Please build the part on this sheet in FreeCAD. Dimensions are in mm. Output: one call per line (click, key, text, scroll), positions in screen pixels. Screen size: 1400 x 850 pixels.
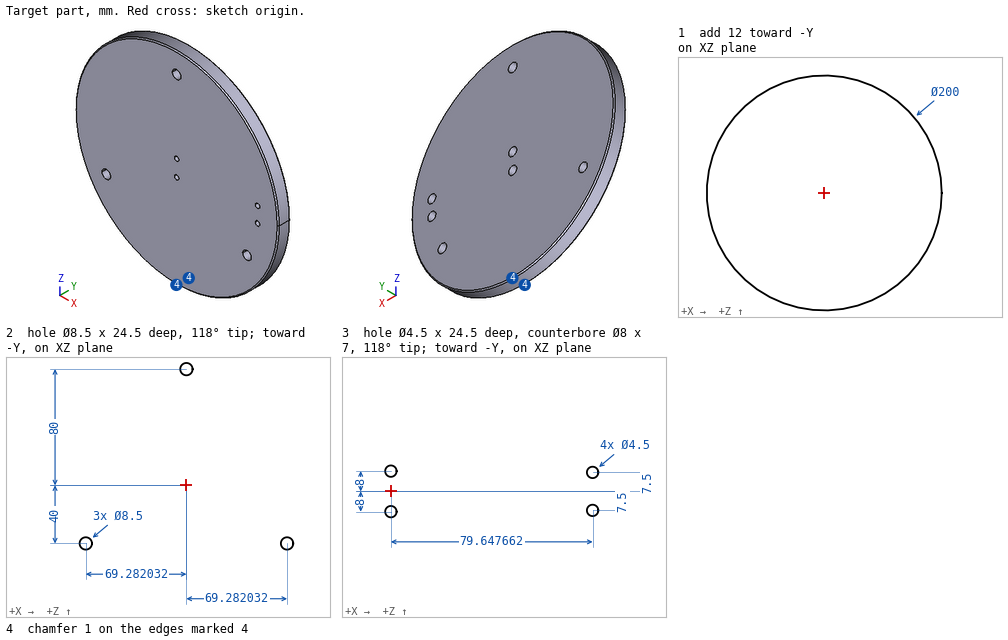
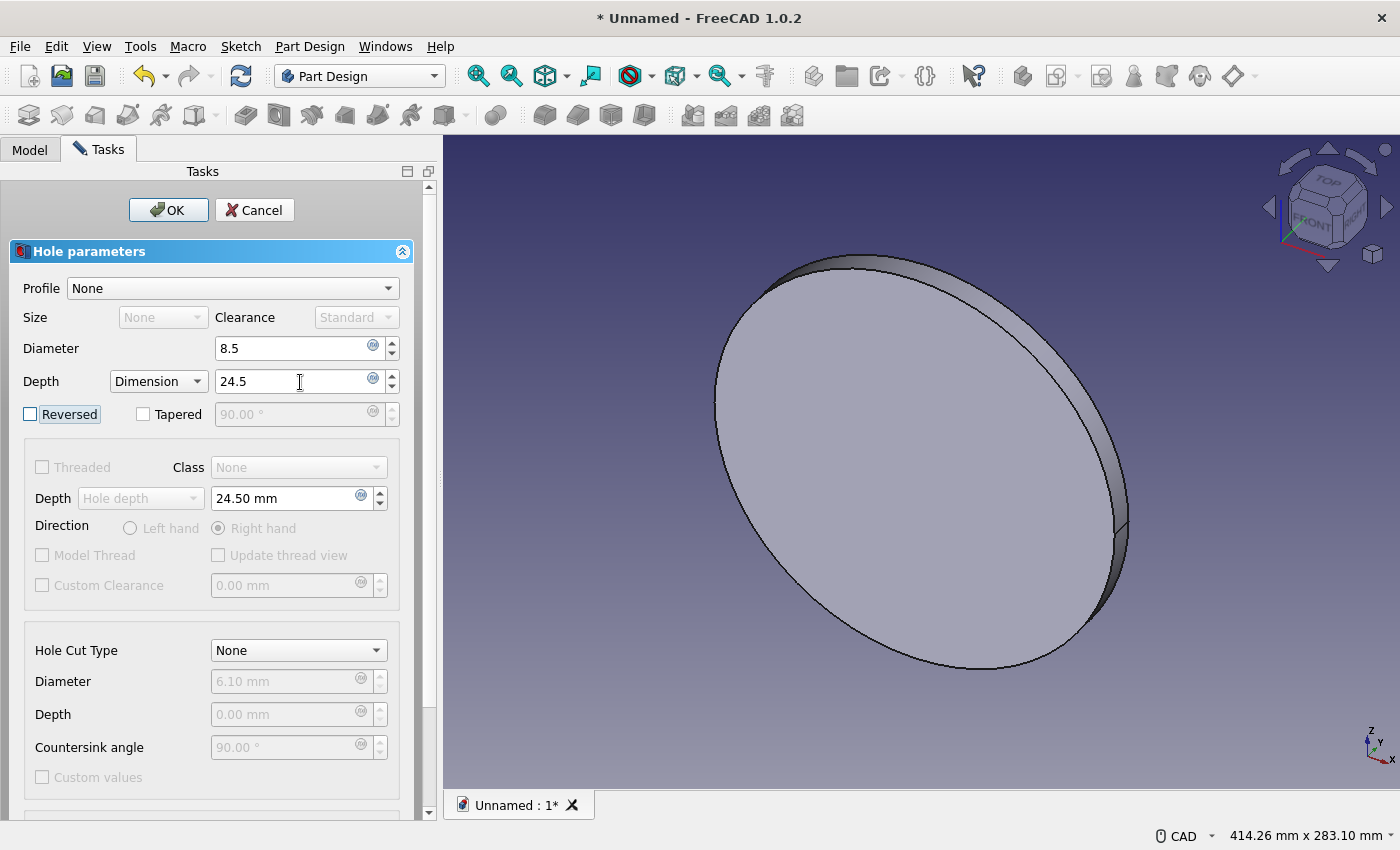
click(31, 414)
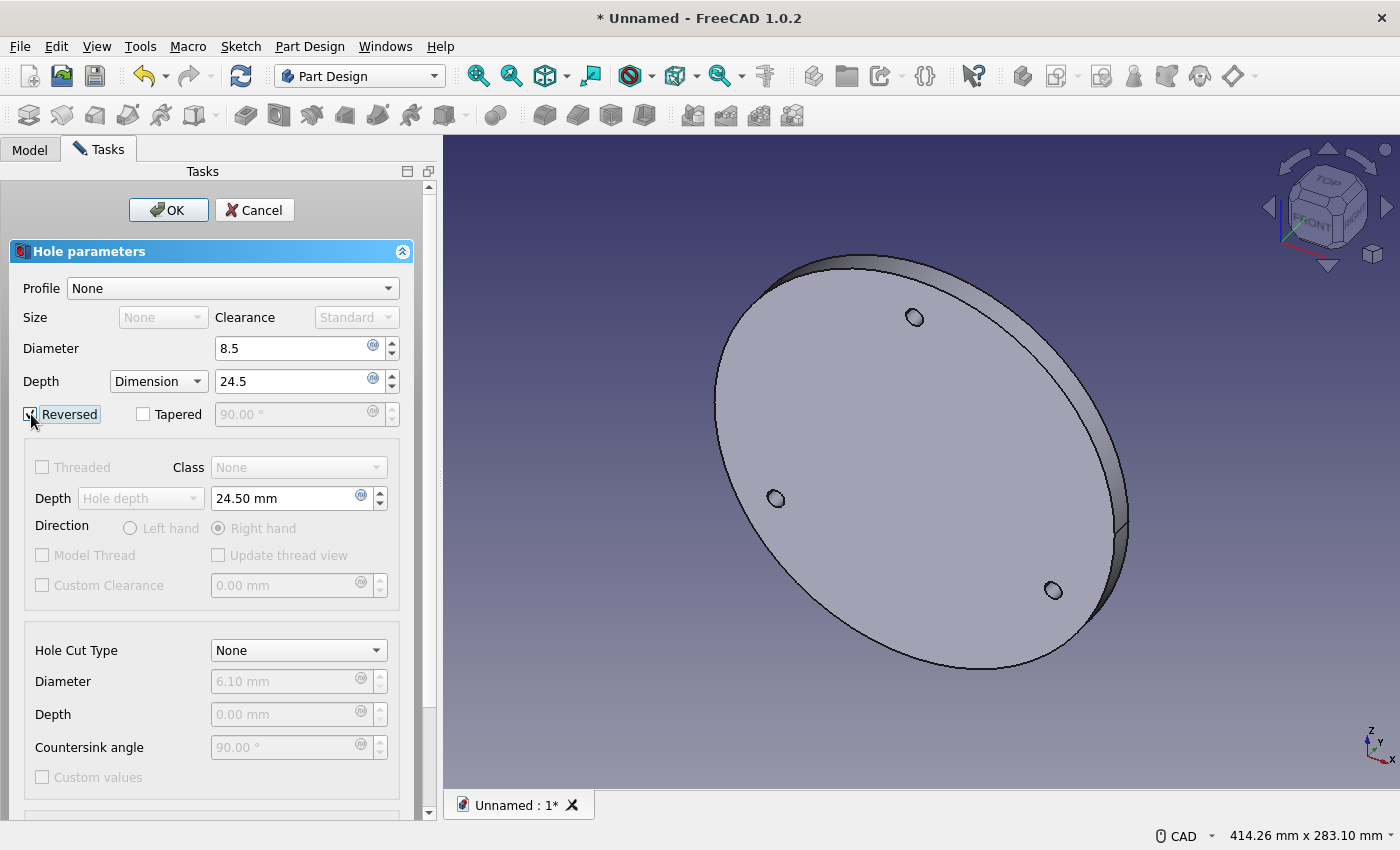
click(169, 210)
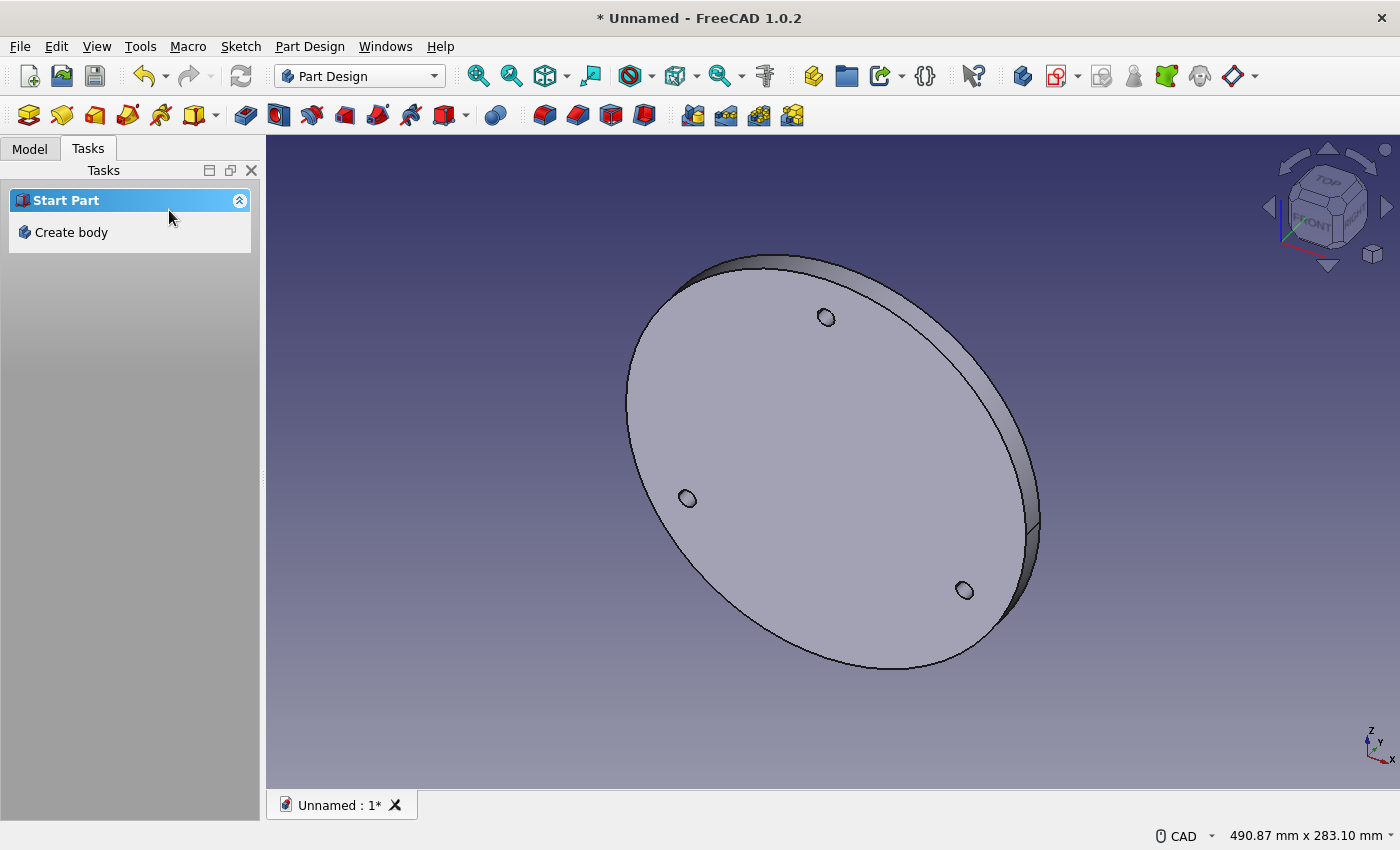
click(1056, 76)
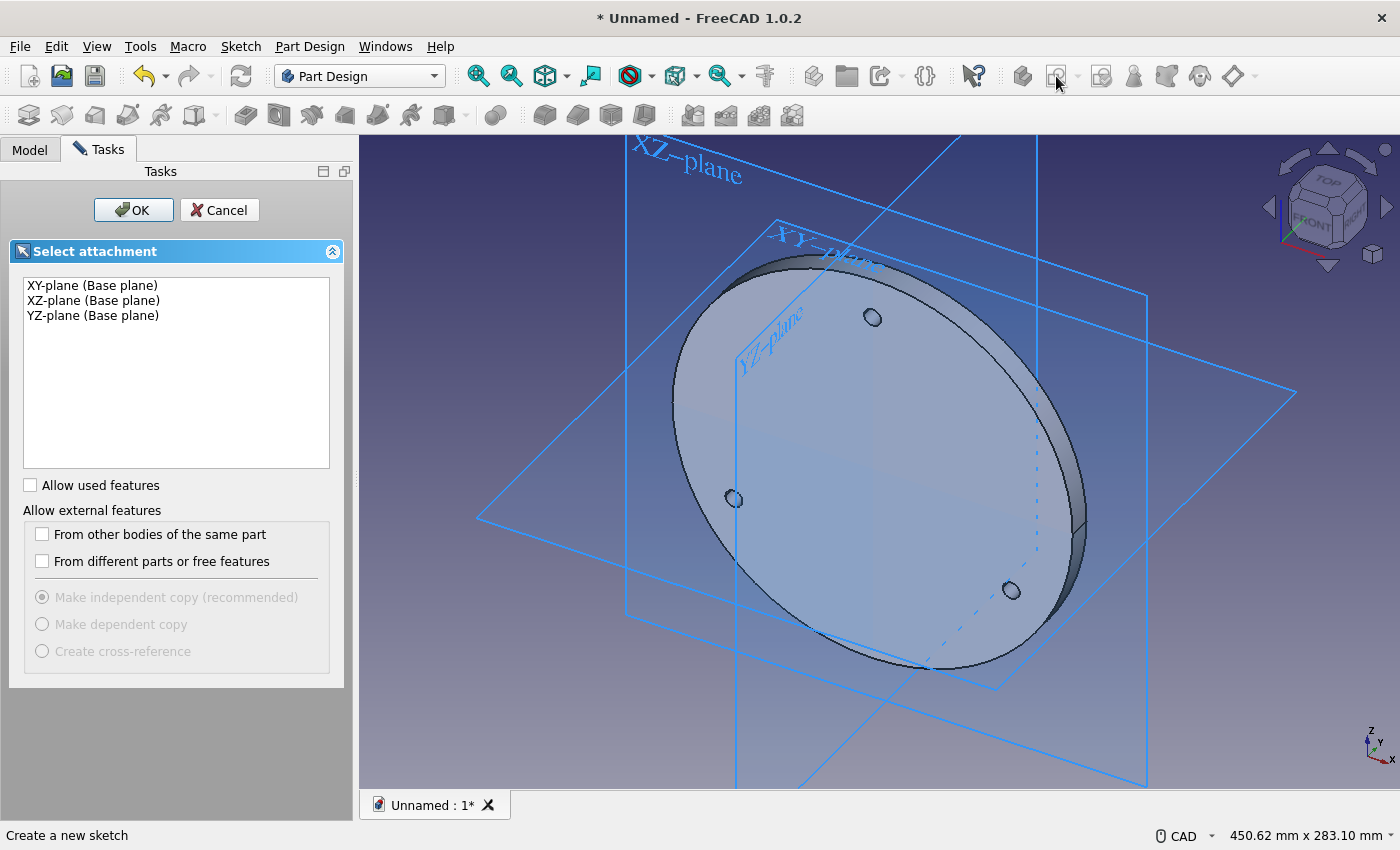
click(84, 300)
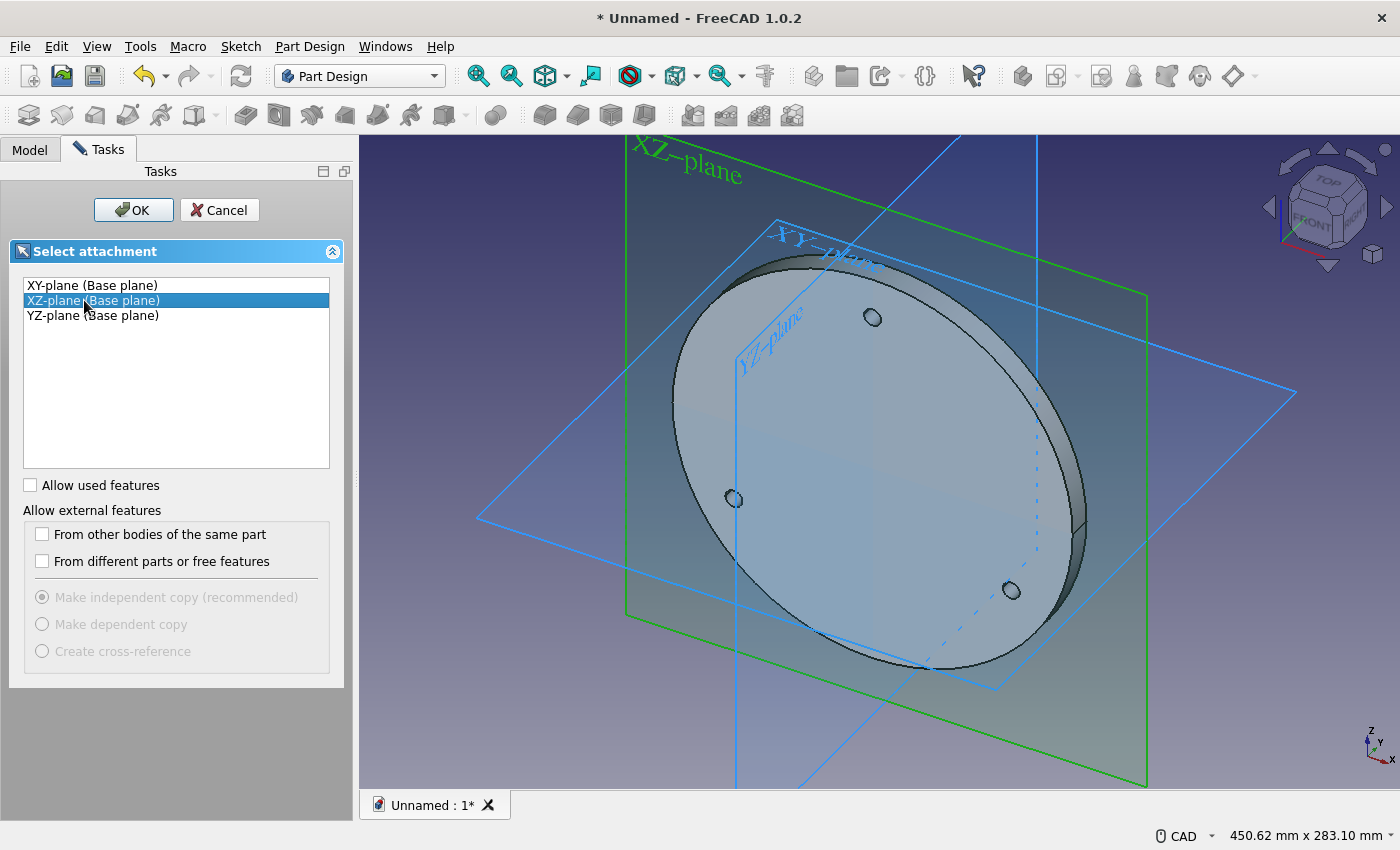
click(134, 210)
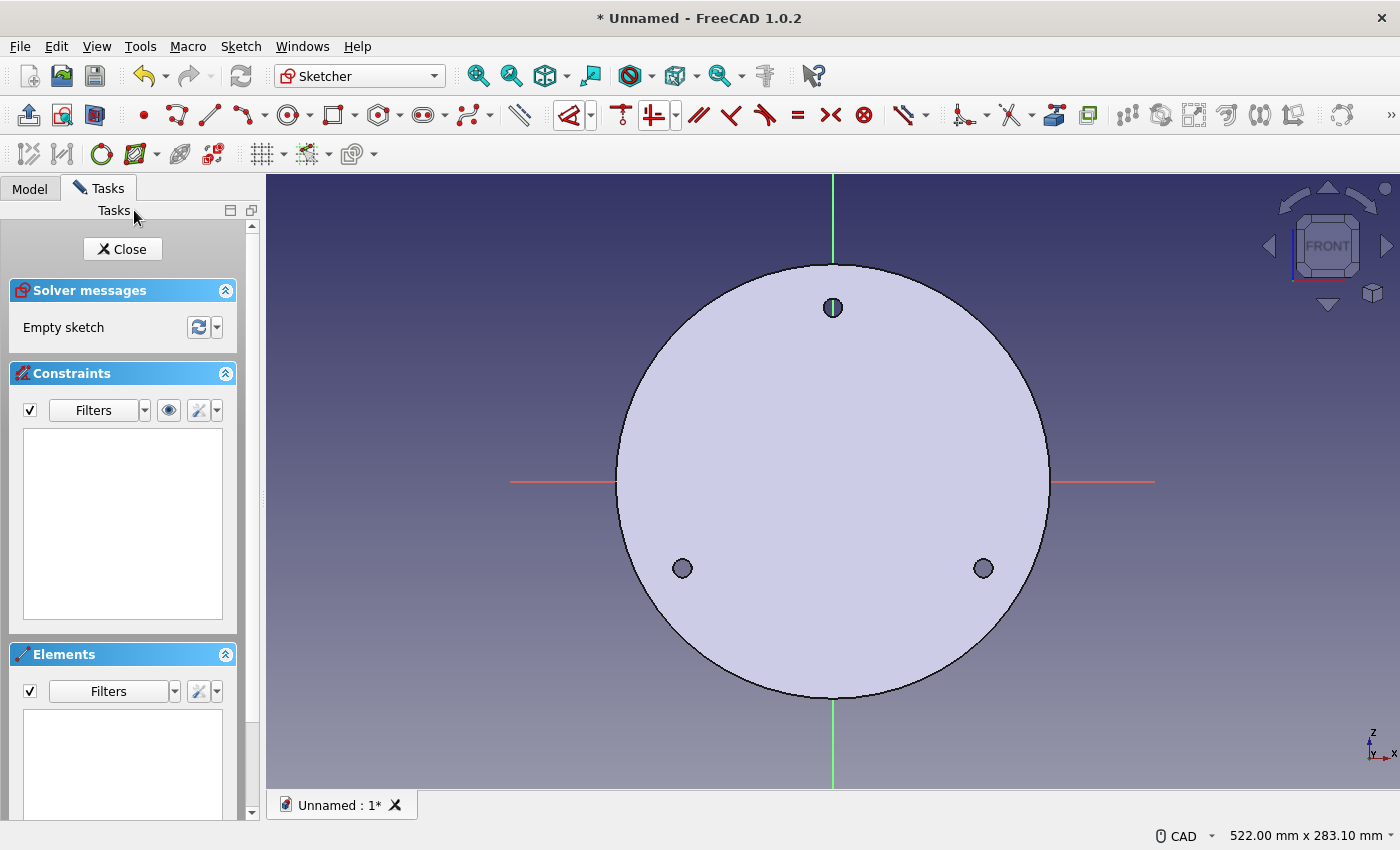
key(q)
key(s)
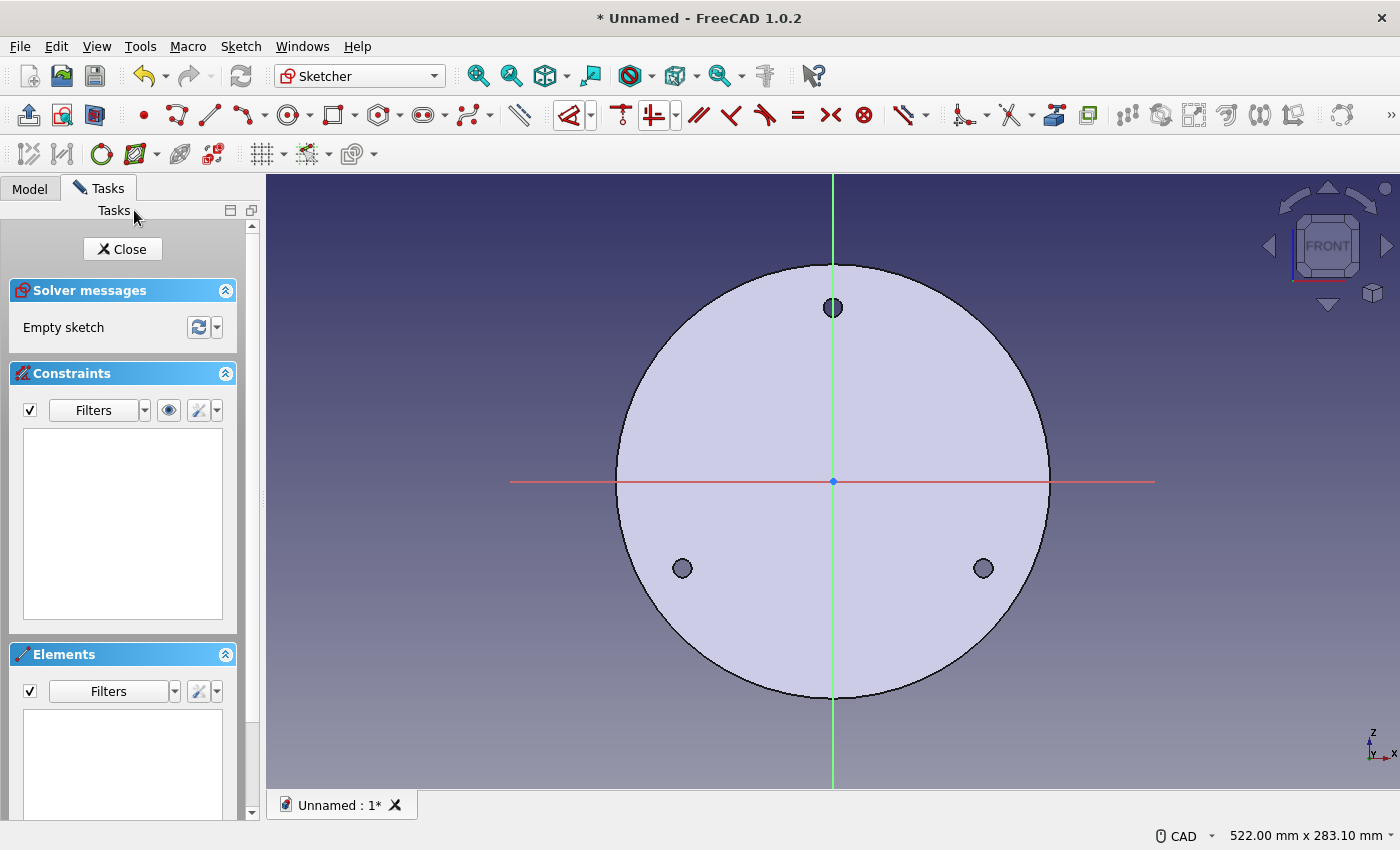
scroll(986, 482, up, 6)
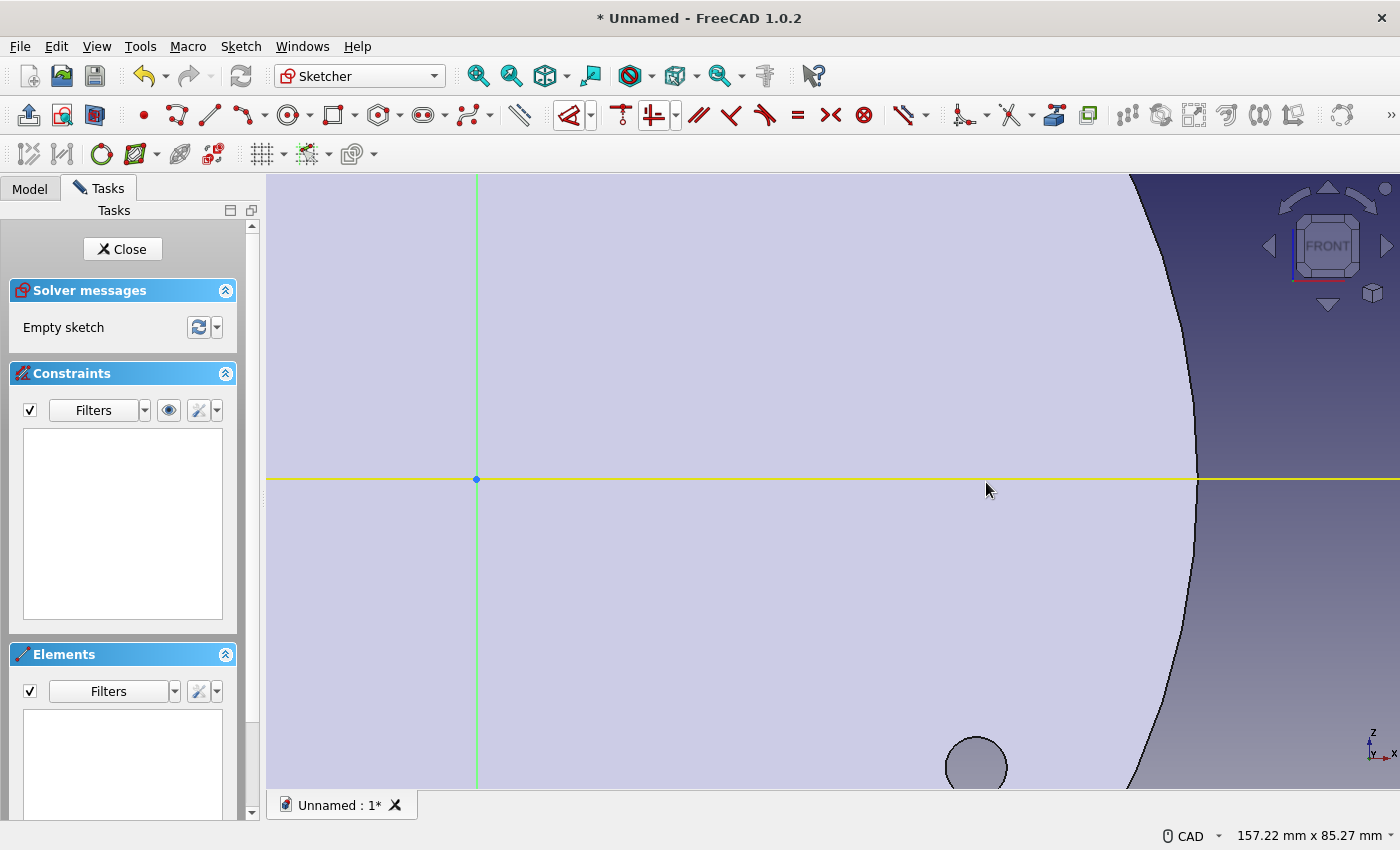
click(288, 116)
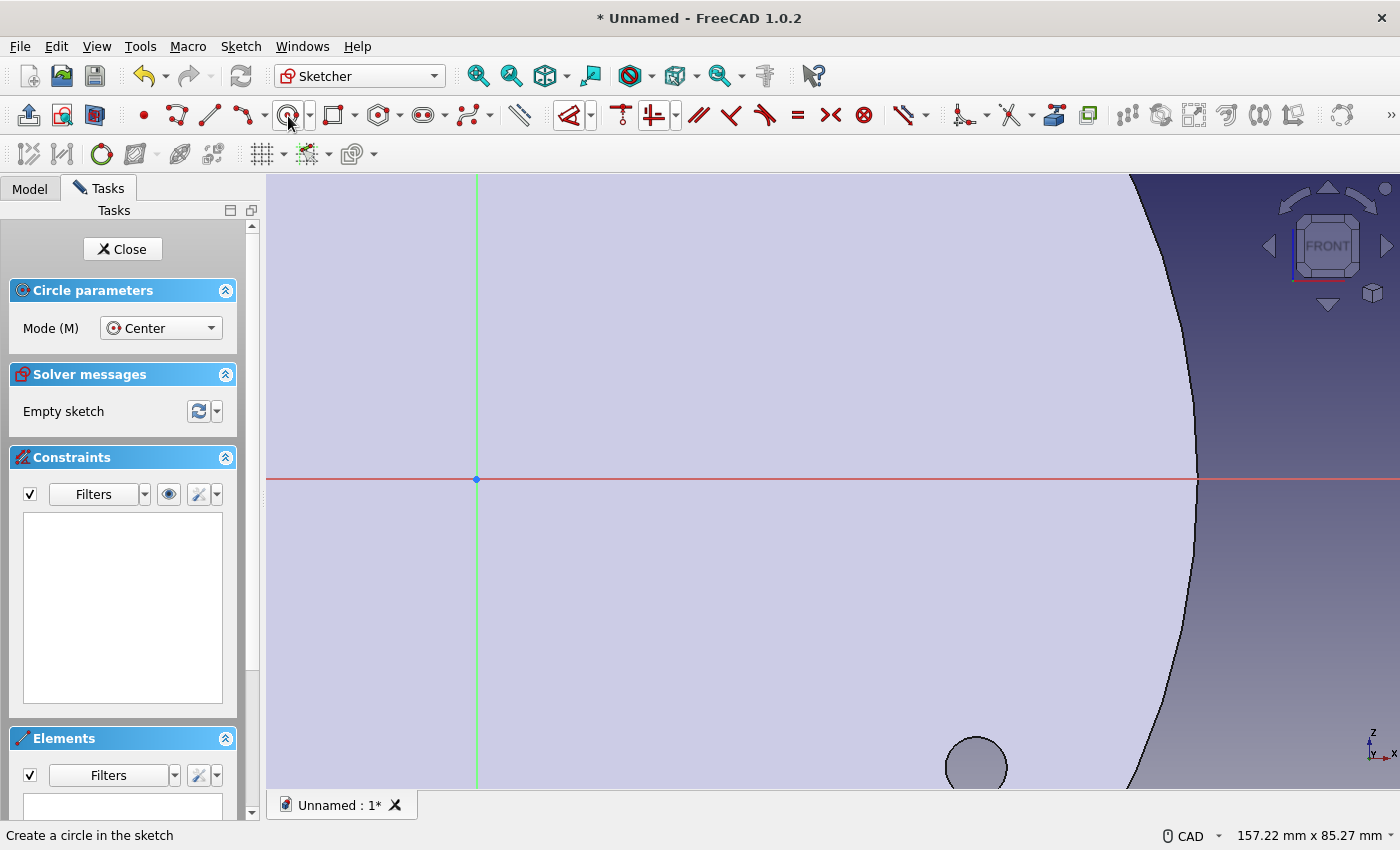
scroll(1051, 533, up, 2)